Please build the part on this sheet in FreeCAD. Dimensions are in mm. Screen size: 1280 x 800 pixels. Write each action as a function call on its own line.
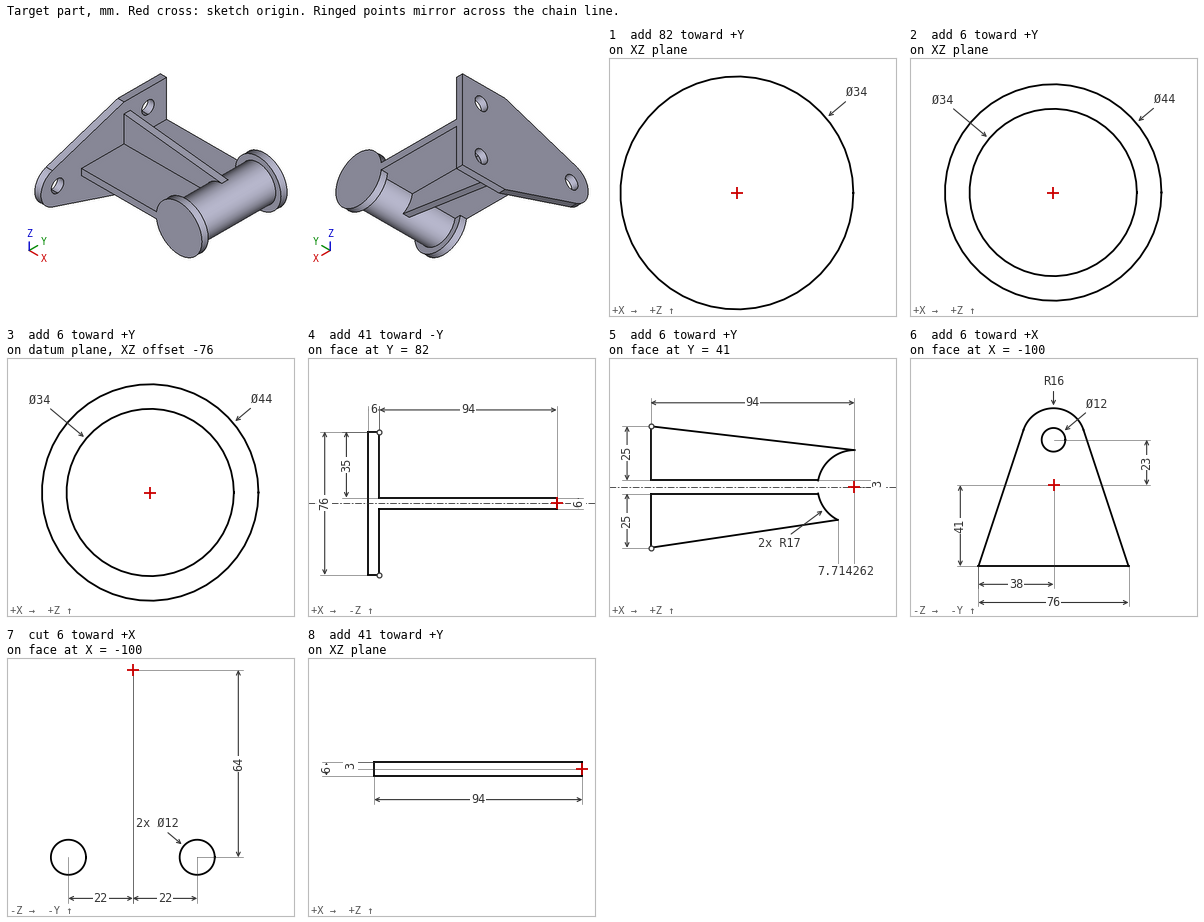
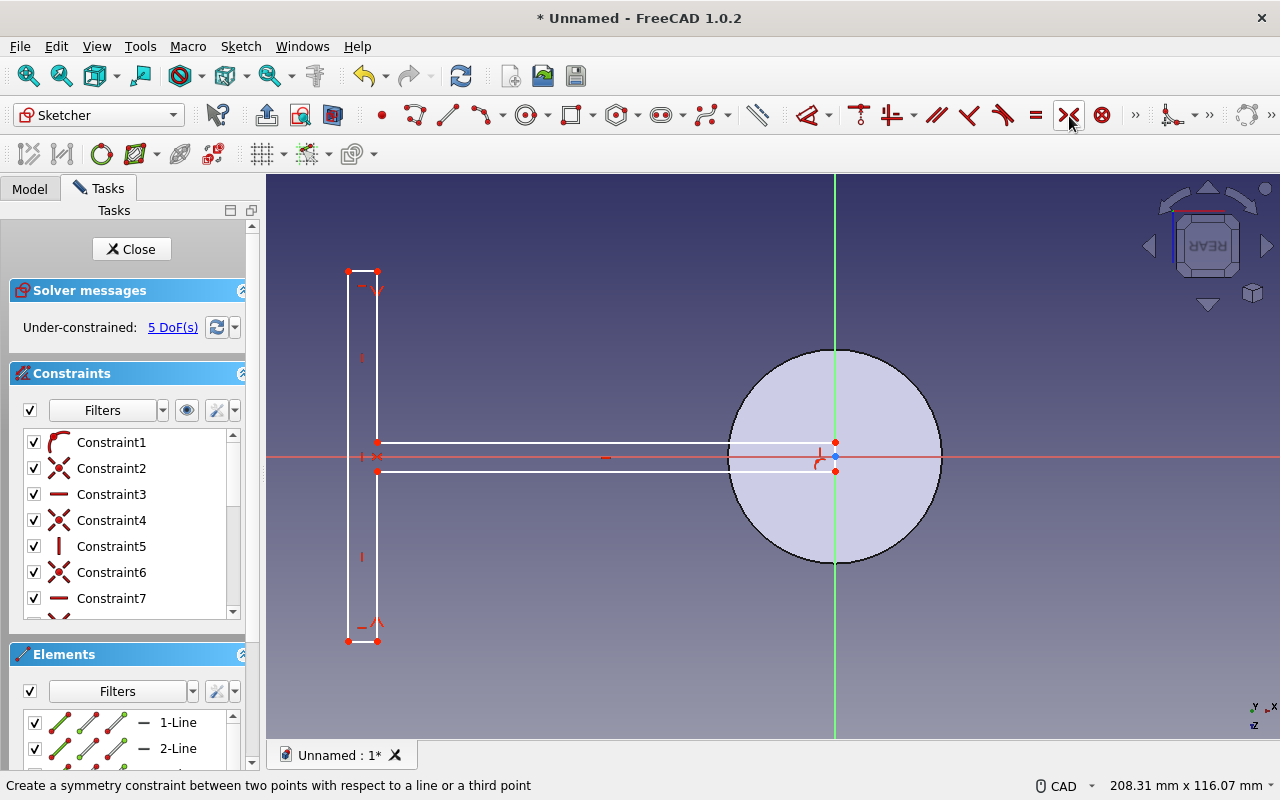
click(806, 116)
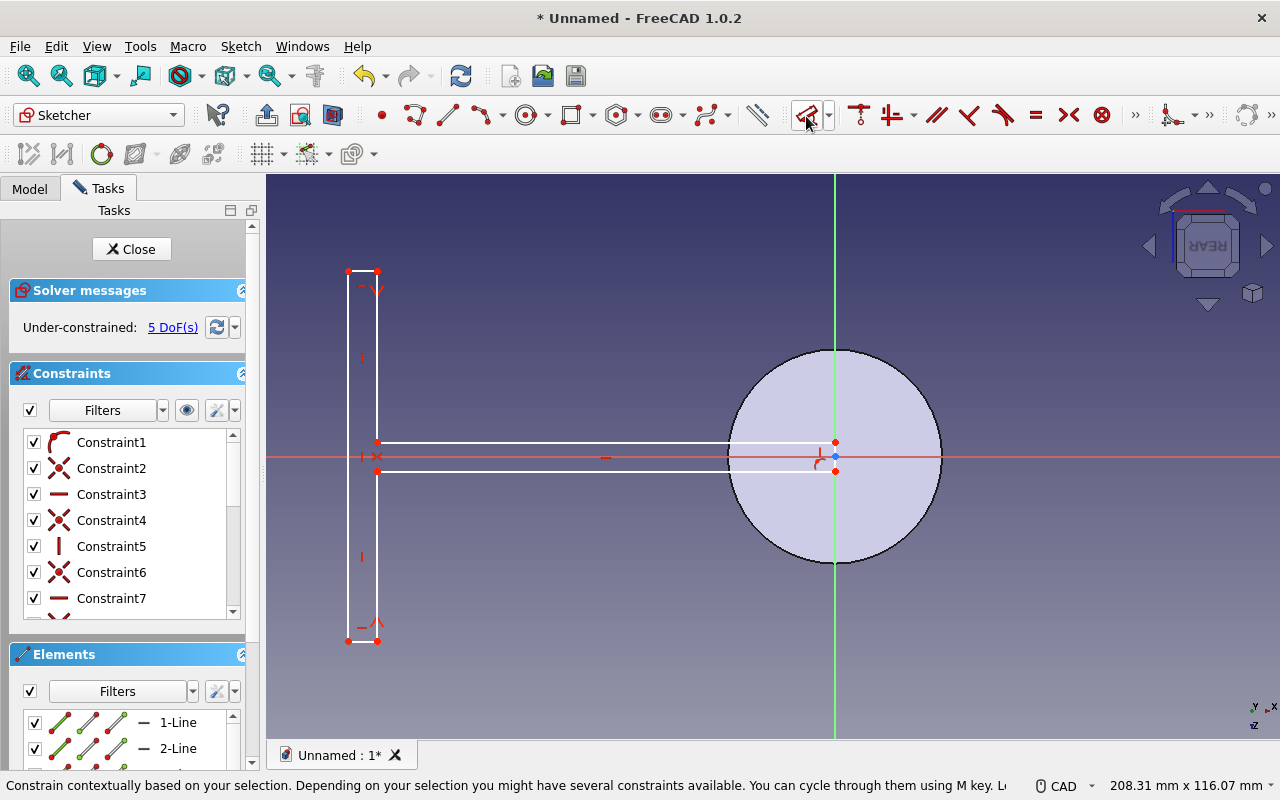
scroll(835, 460, up, 2)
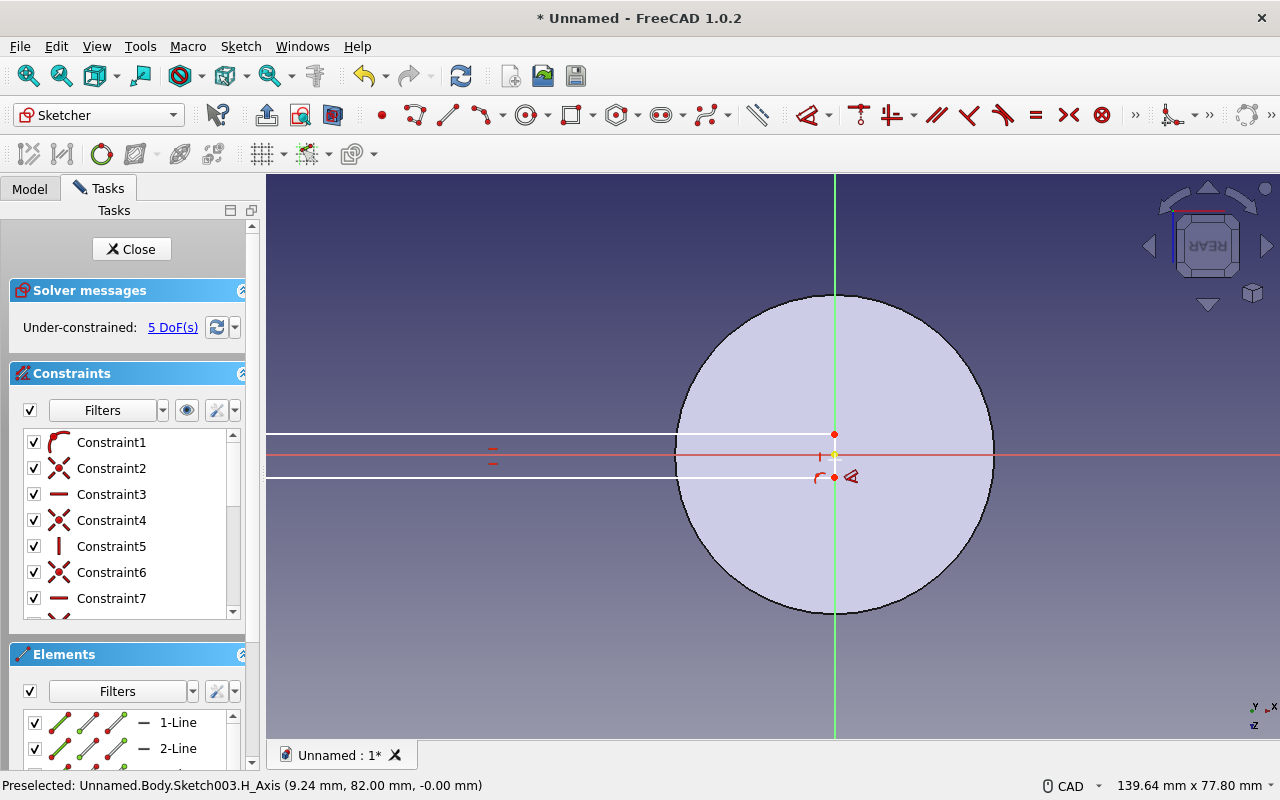
click(835, 460)
click(869, 441)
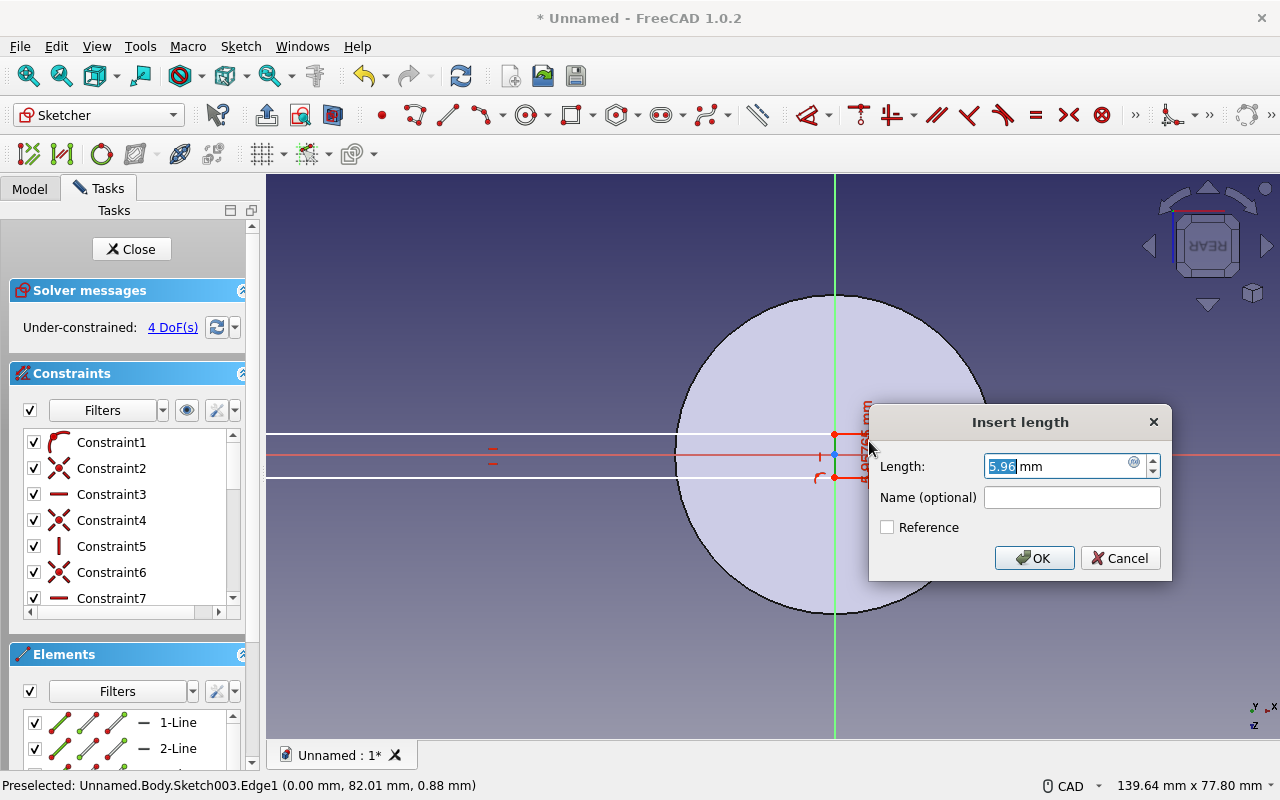
text(6)
key(Return)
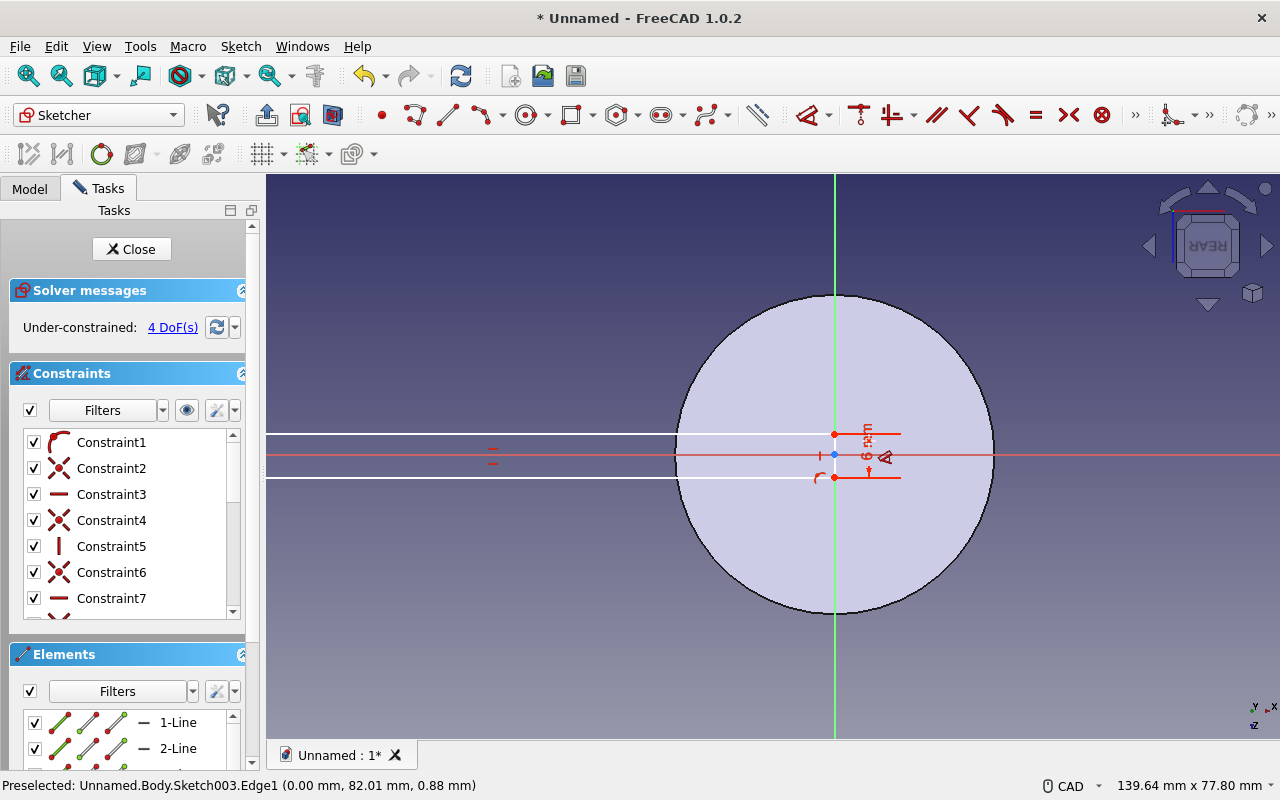
scroll(1115, 460, down, 2)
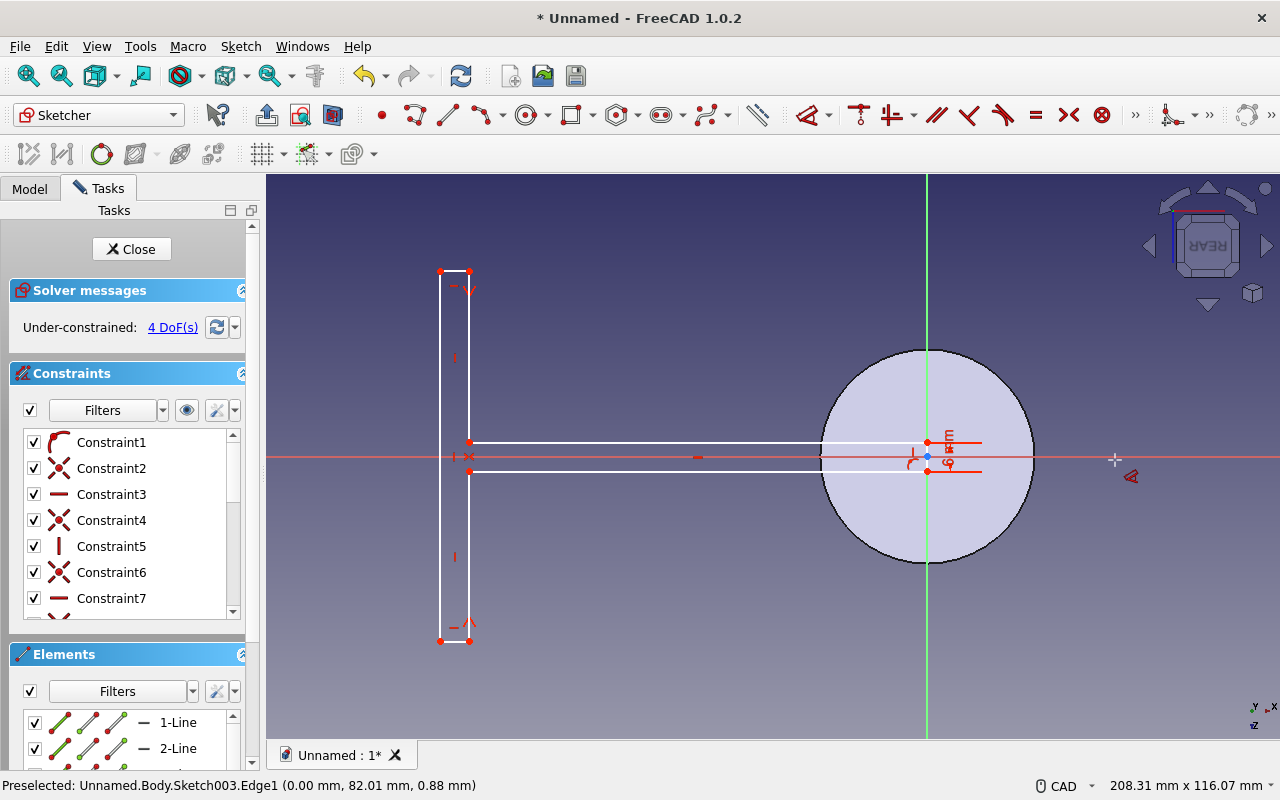
scroll(461, 271, up, 3)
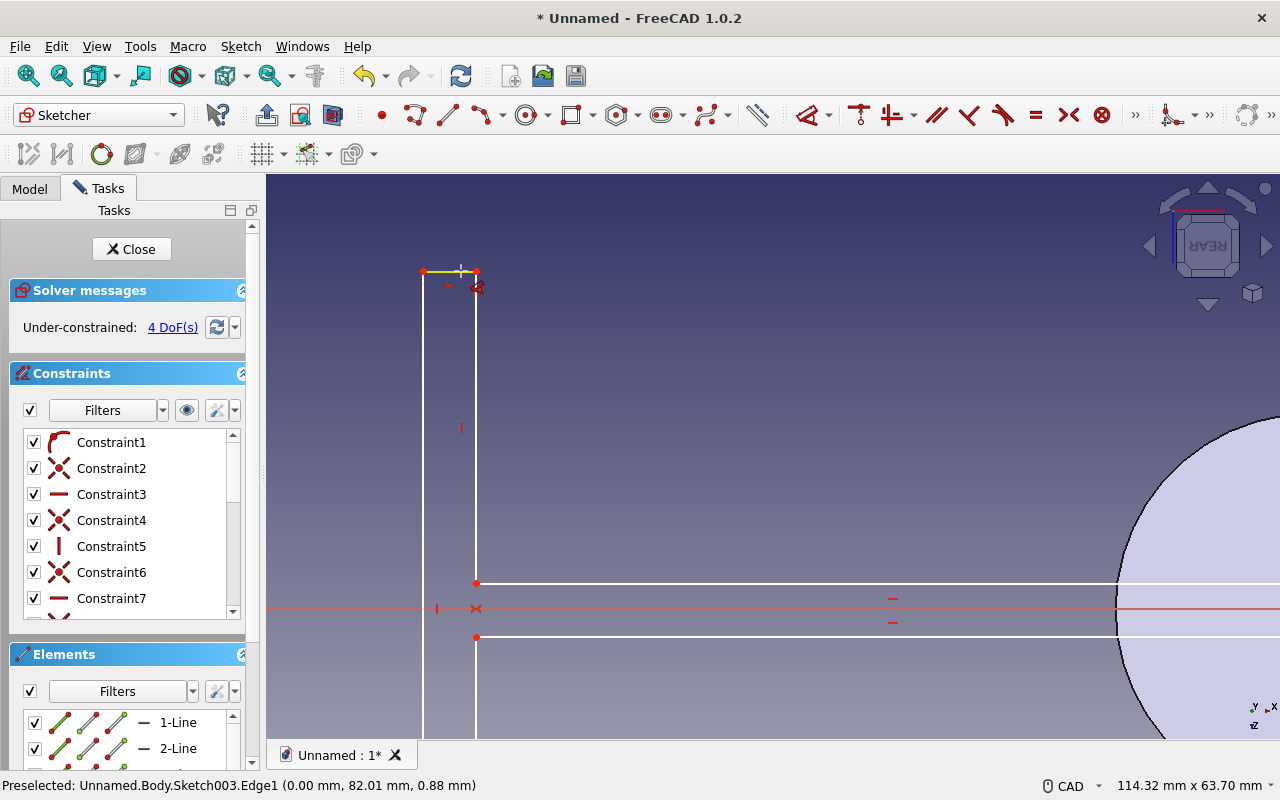
click(460, 272)
click(450, 238)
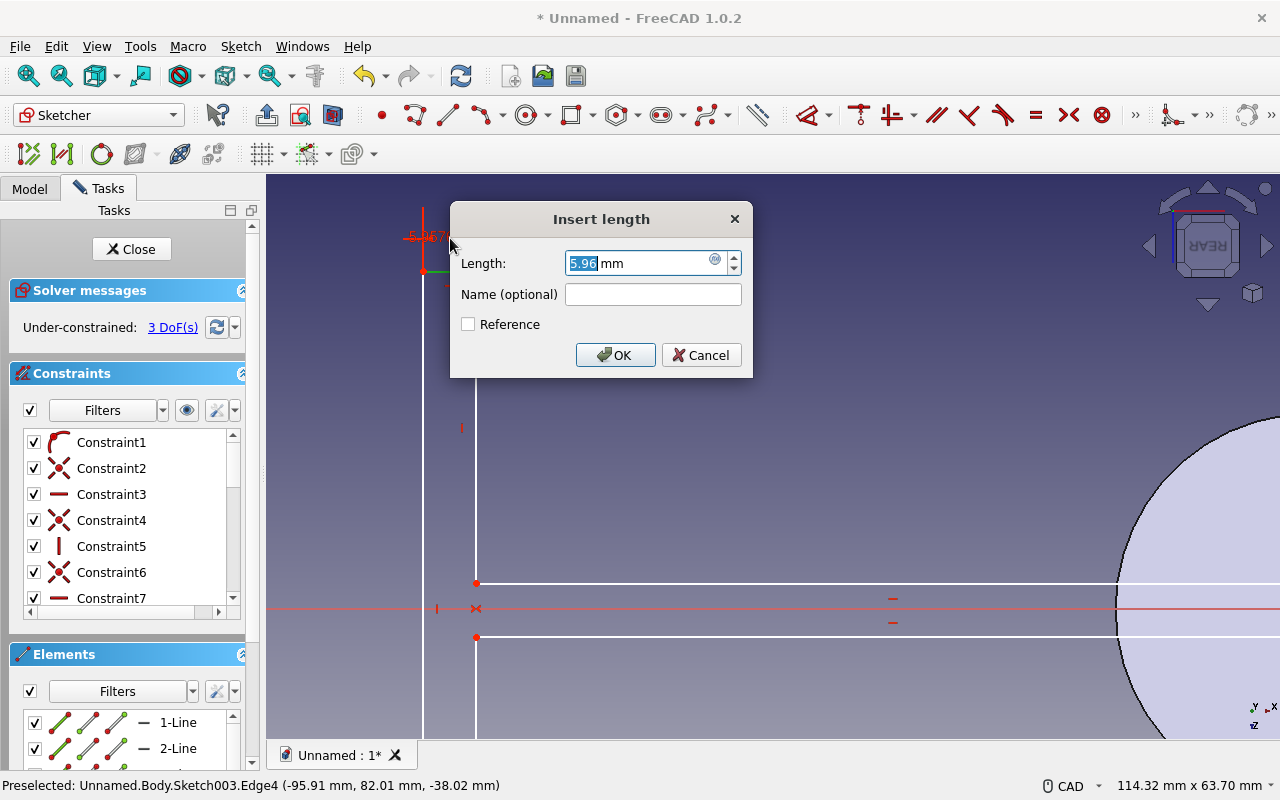
text(6)
key(Return)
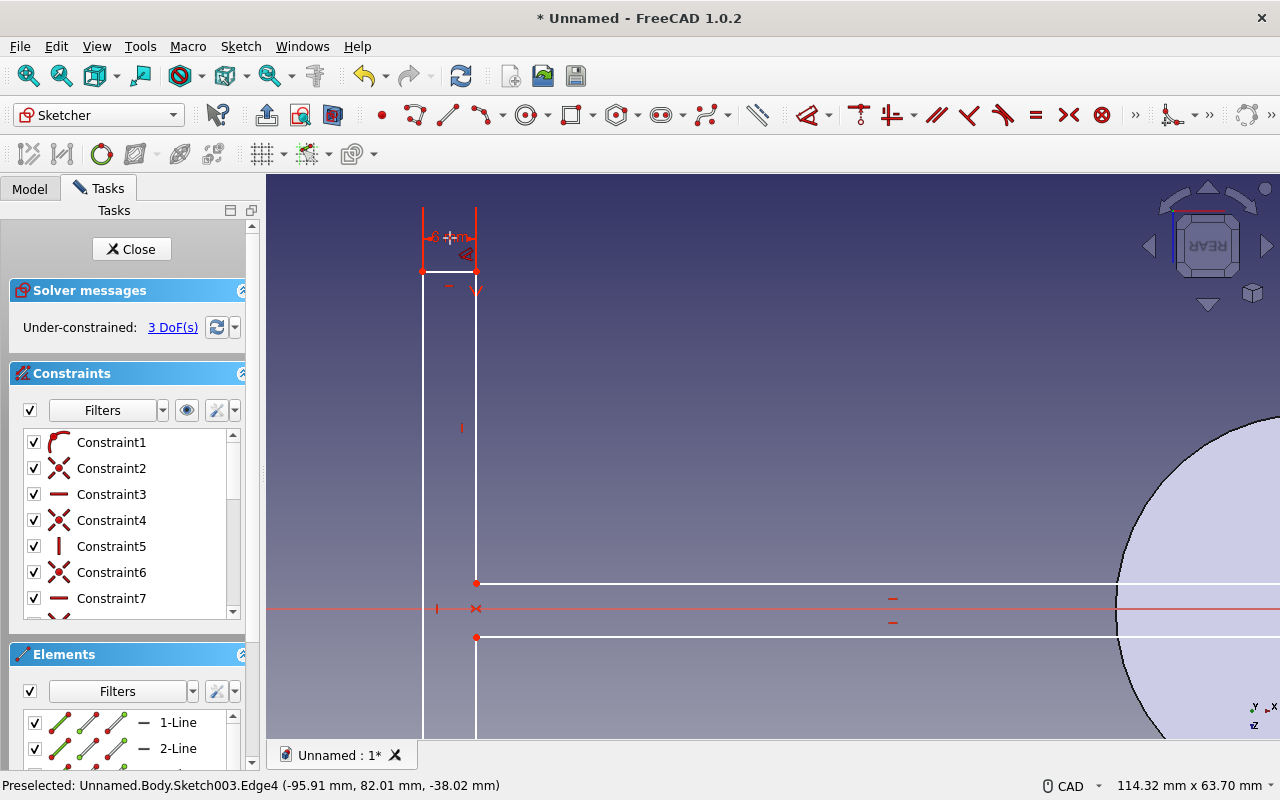
click(1060, 584)
click(796, 550)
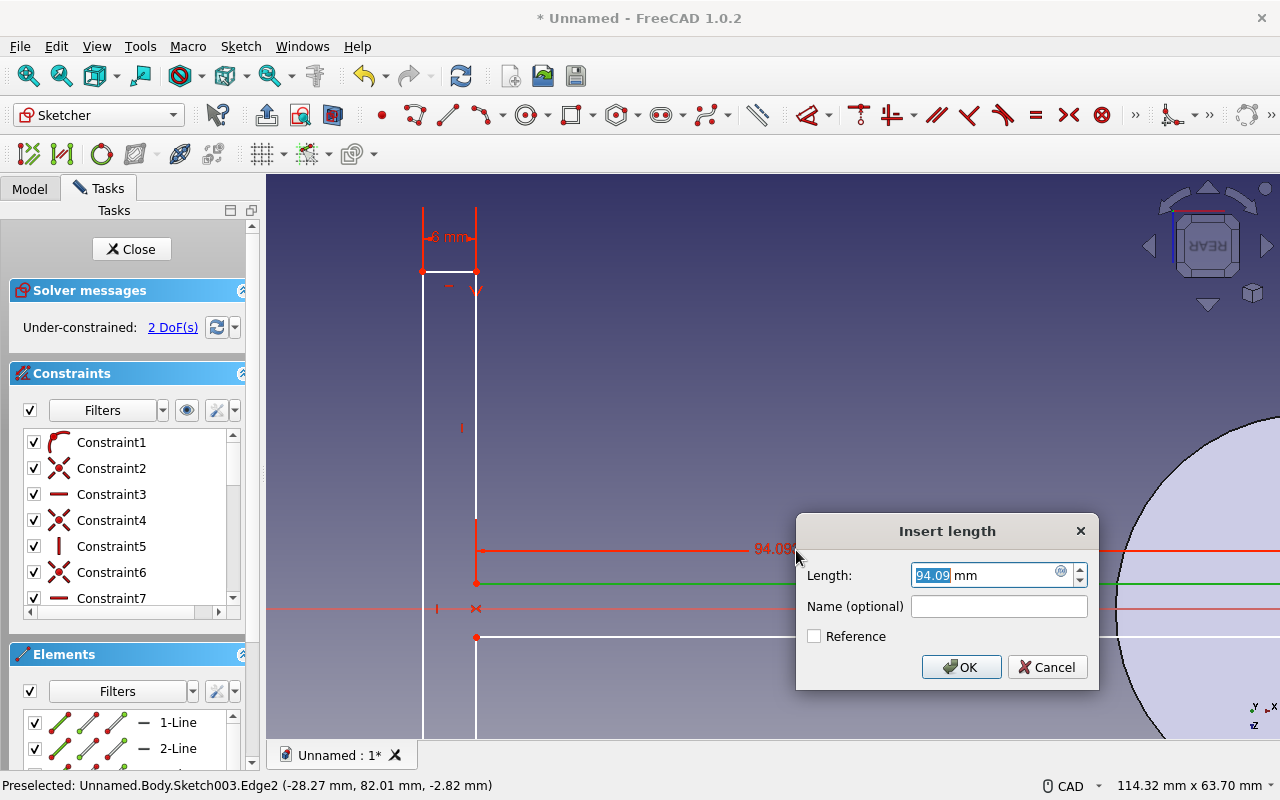
text(94)
key(Return)